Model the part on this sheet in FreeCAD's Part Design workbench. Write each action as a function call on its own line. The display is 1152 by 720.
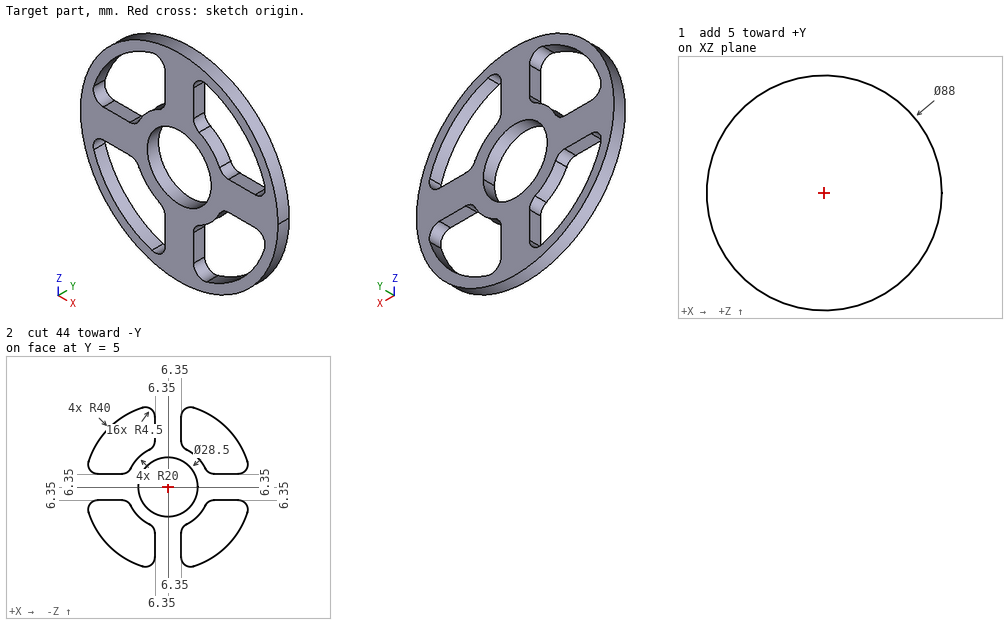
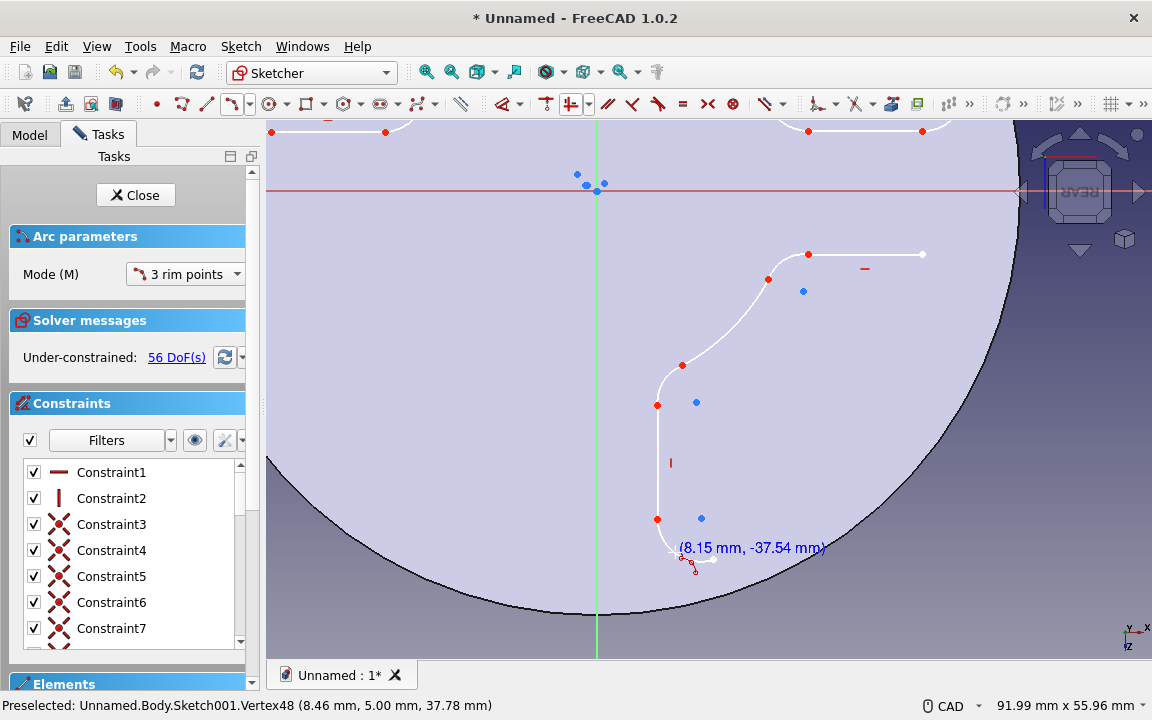
click(713, 560)
click(963, 309)
click(869, 464)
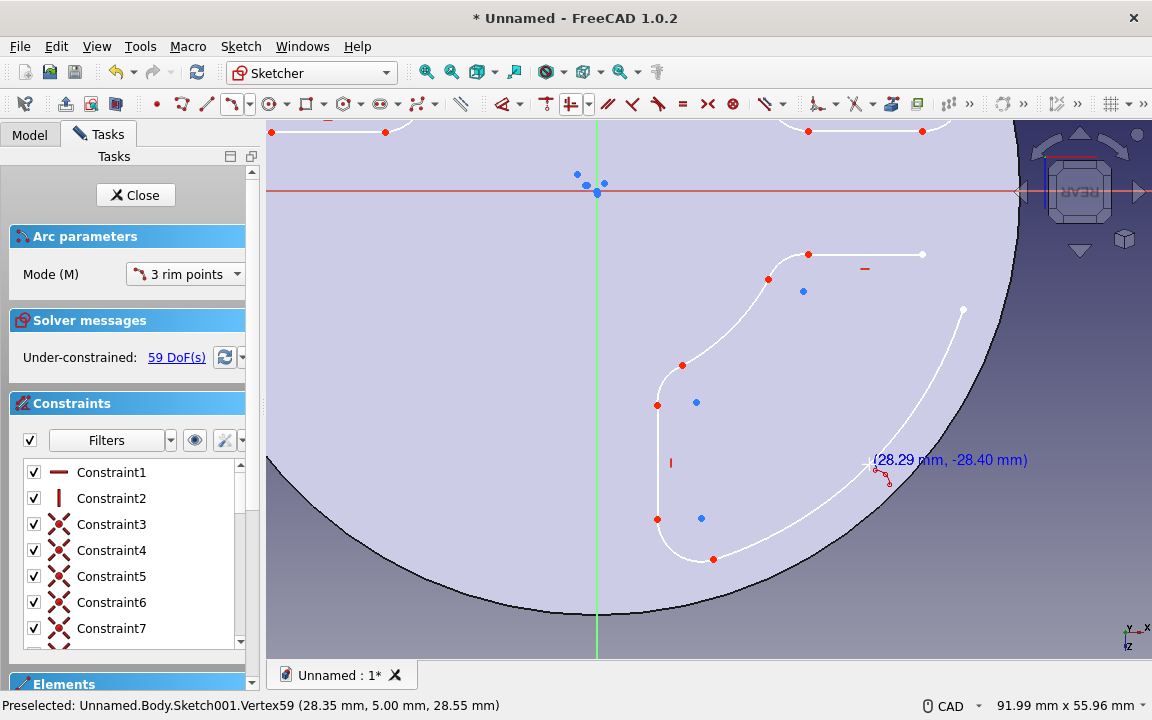
click(963, 310)
click(922, 255)
click(957, 270)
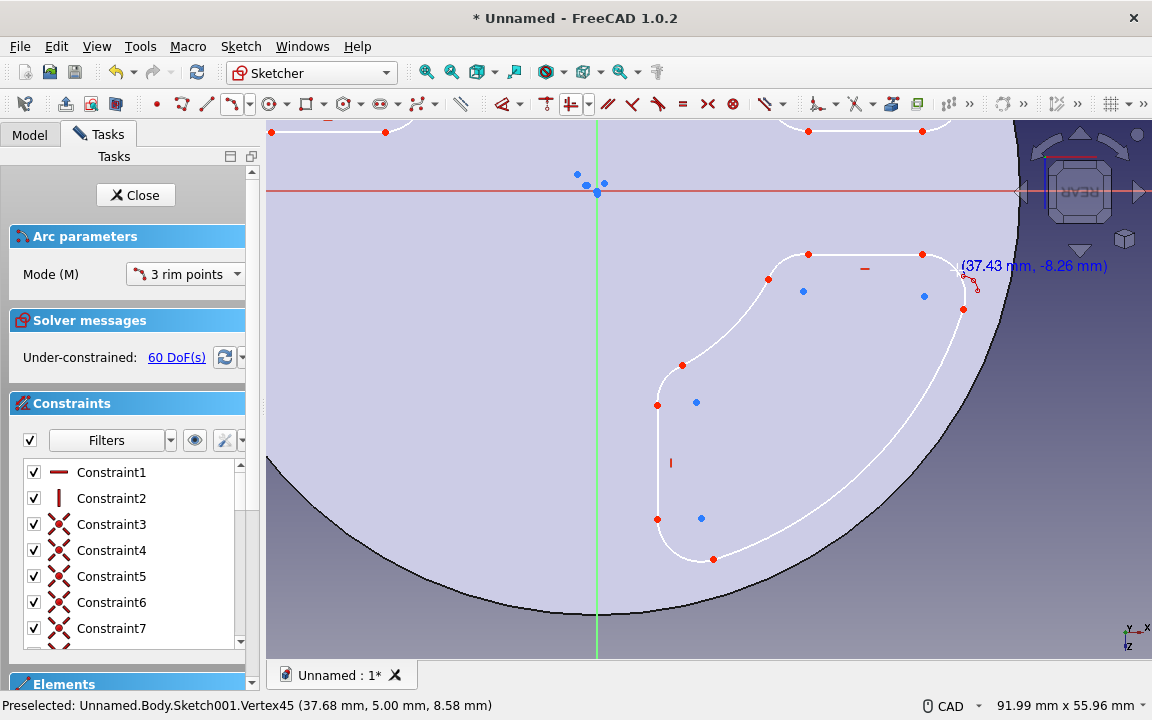
click(207, 104)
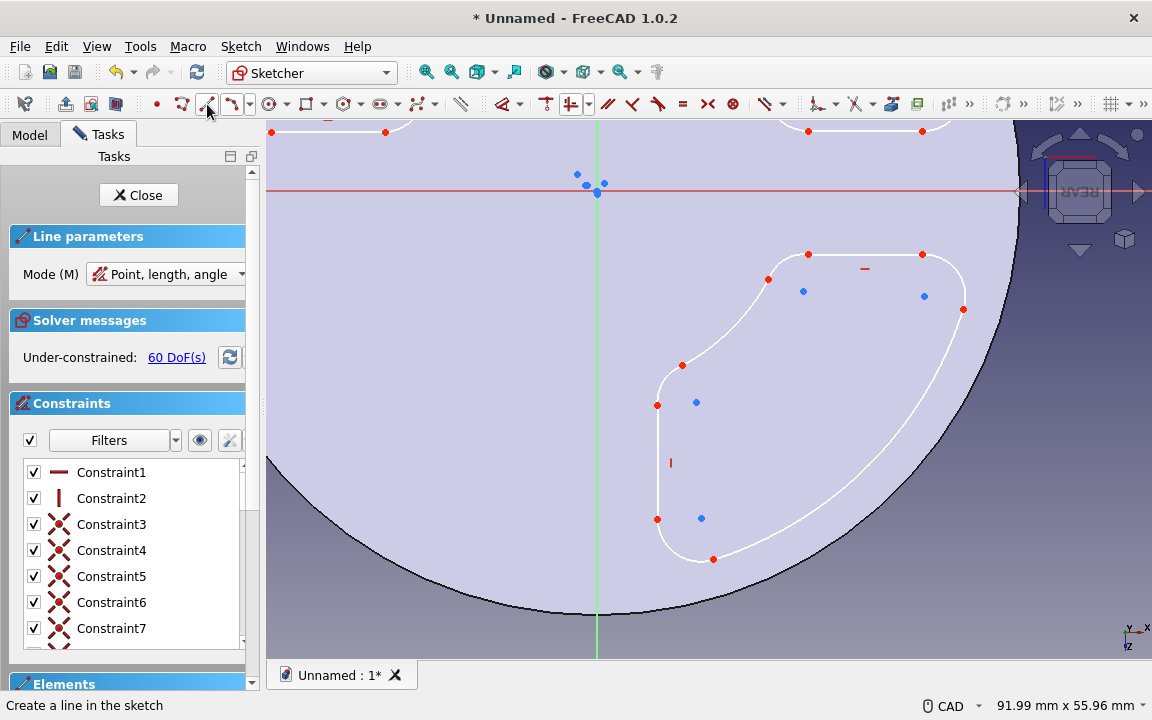
click(535, 517)
click(535, 403)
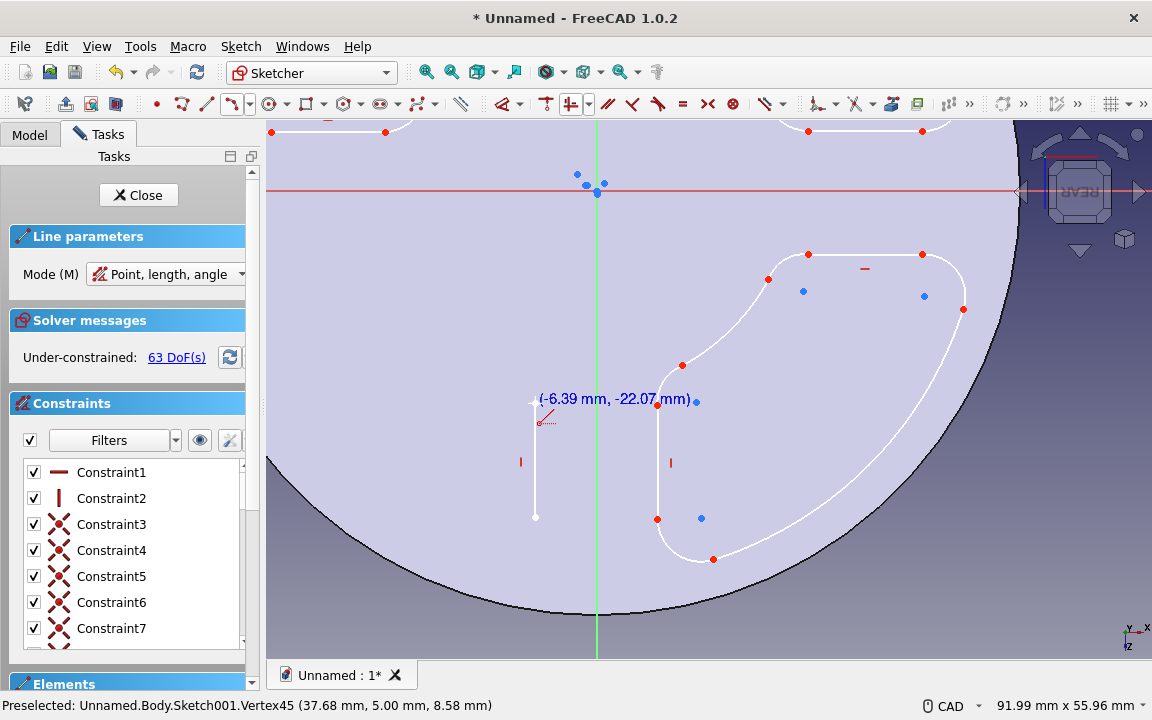
click(385, 253)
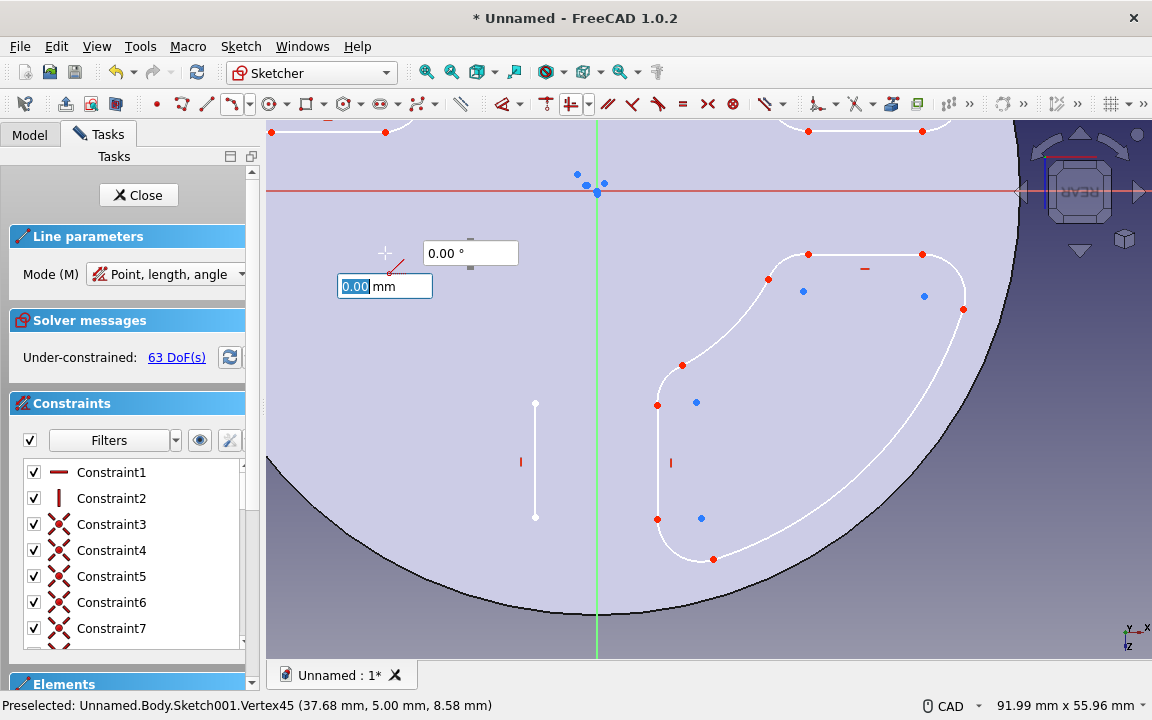
scroll(676, 551, down, 4)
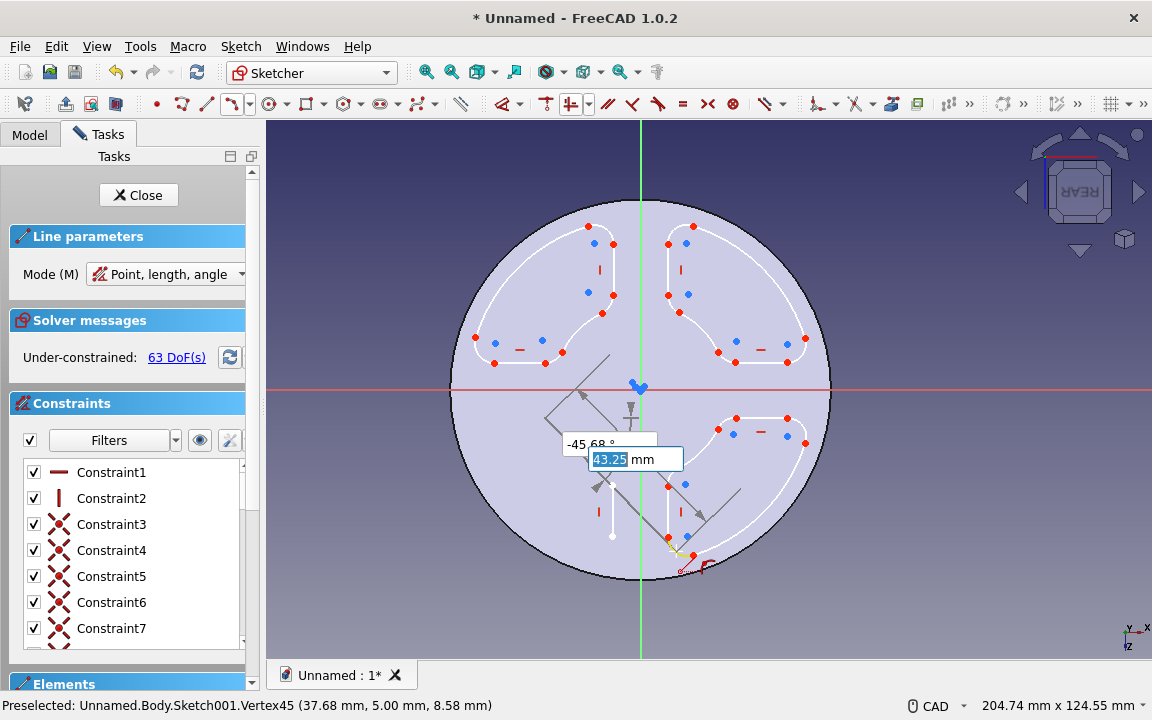
click(494, 418)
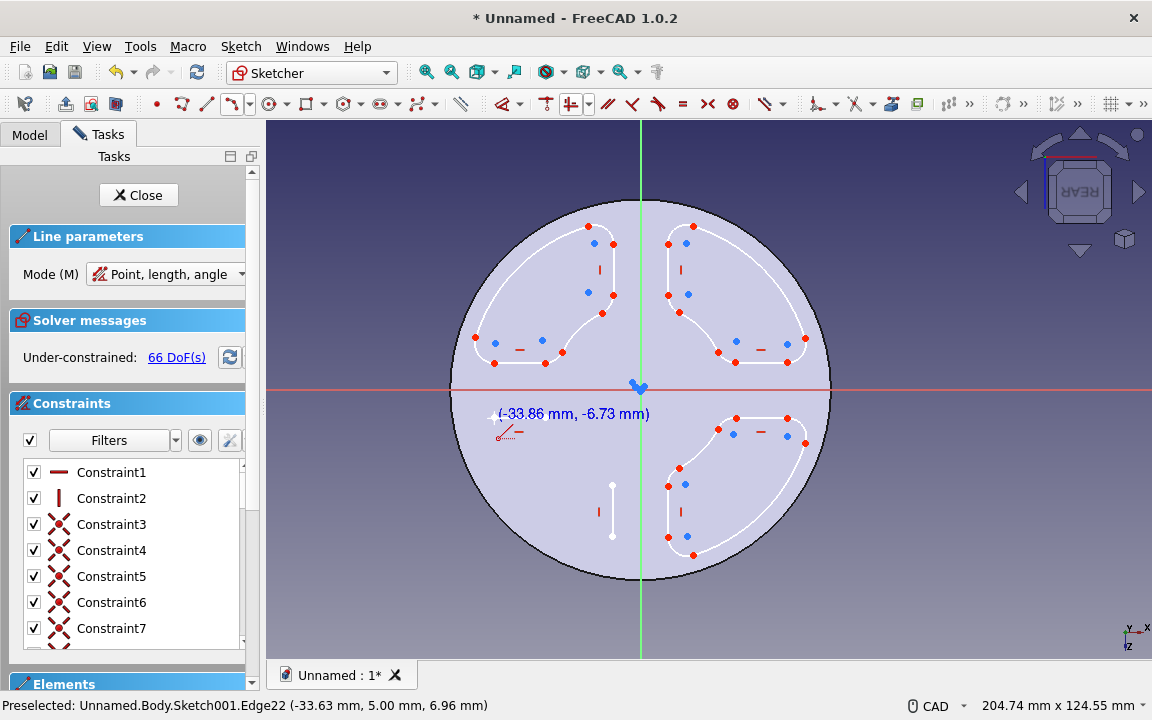
key(g)
key(3)
key(a)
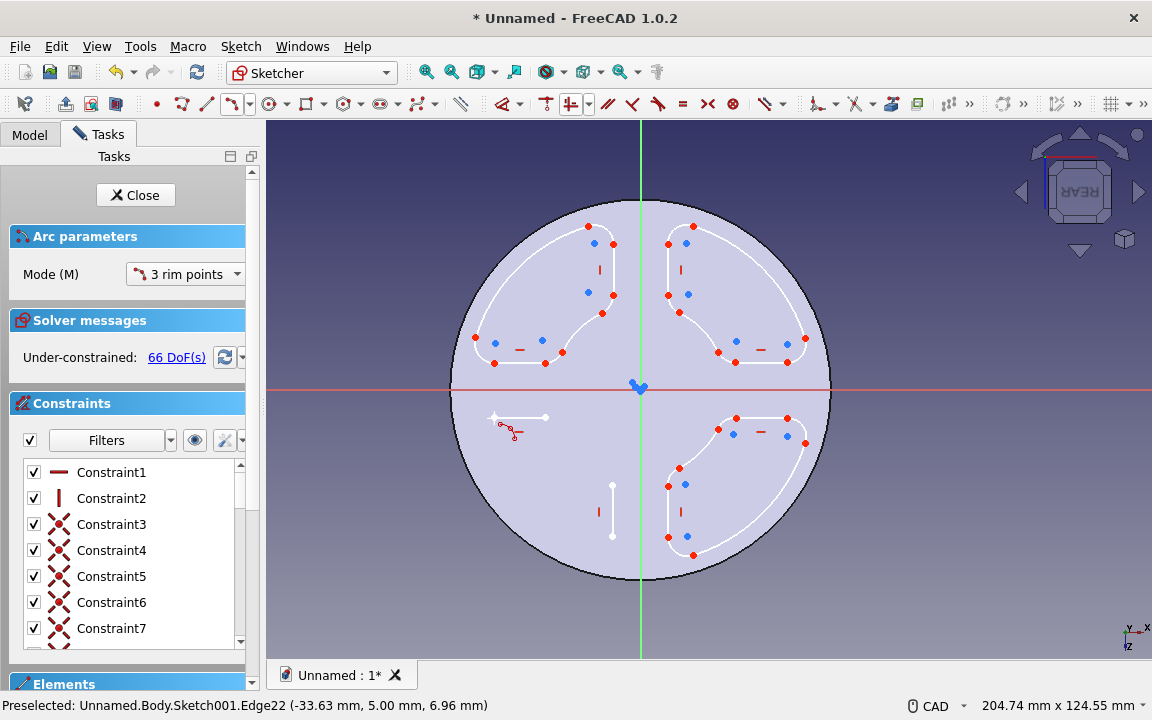
click(613, 485)
click(602, 467)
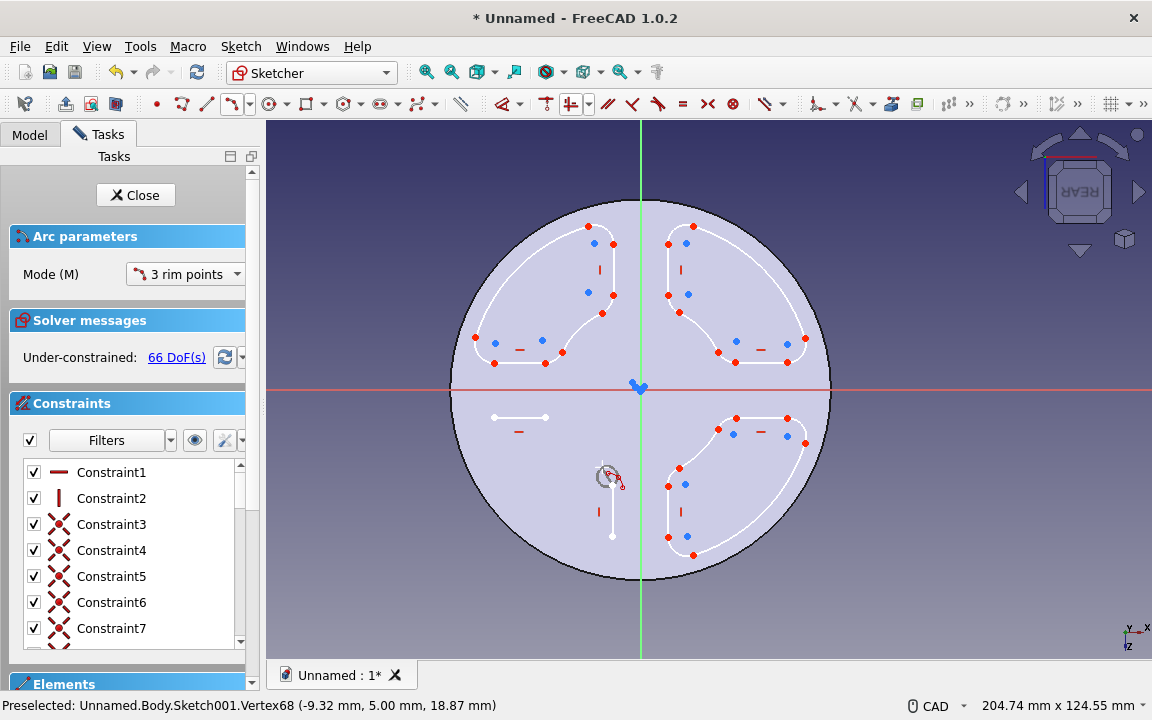
scroll(610, 475, up, 9)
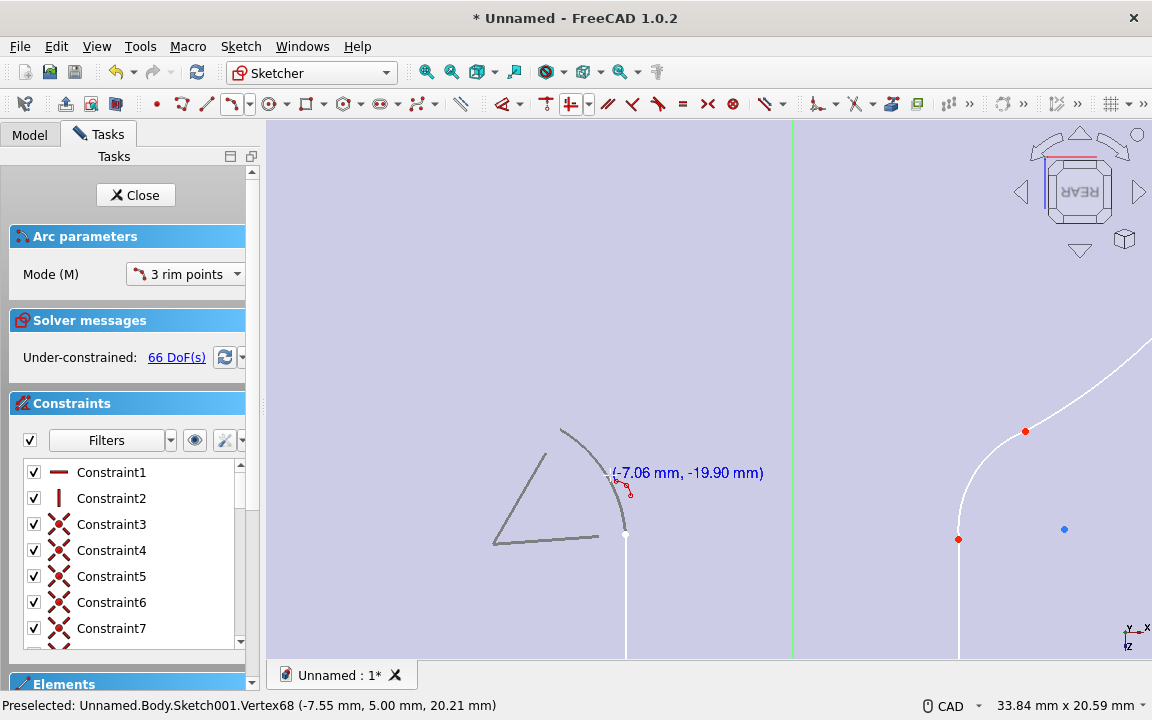
click(609, 470)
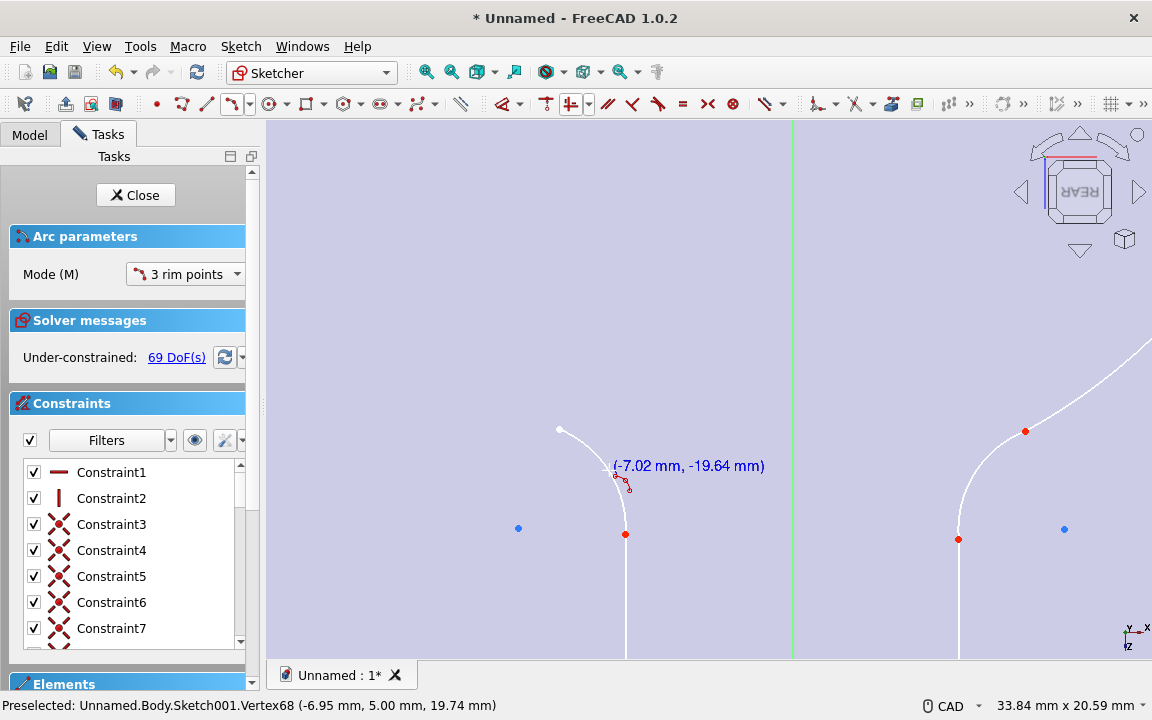
scroll(610, 475, down, 9)